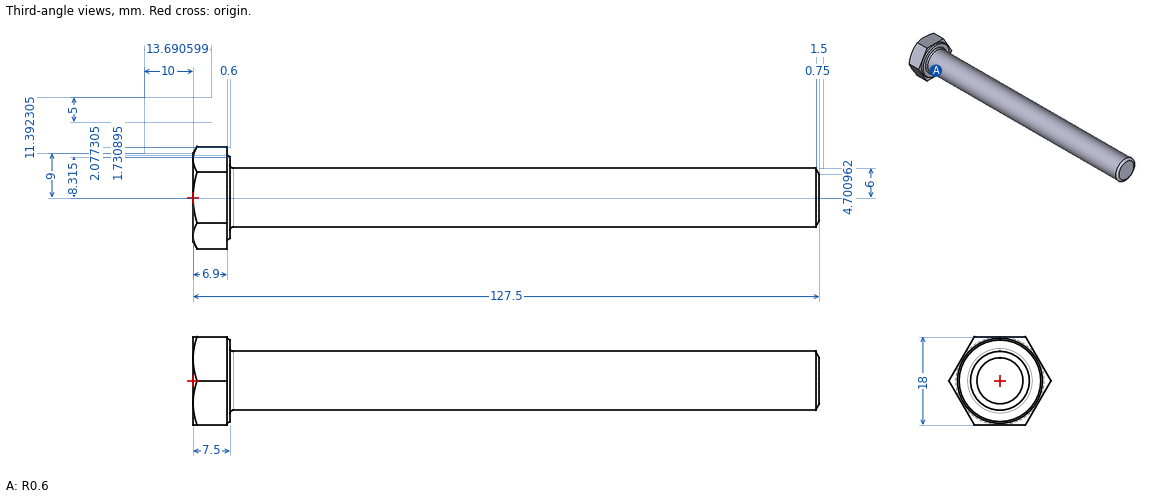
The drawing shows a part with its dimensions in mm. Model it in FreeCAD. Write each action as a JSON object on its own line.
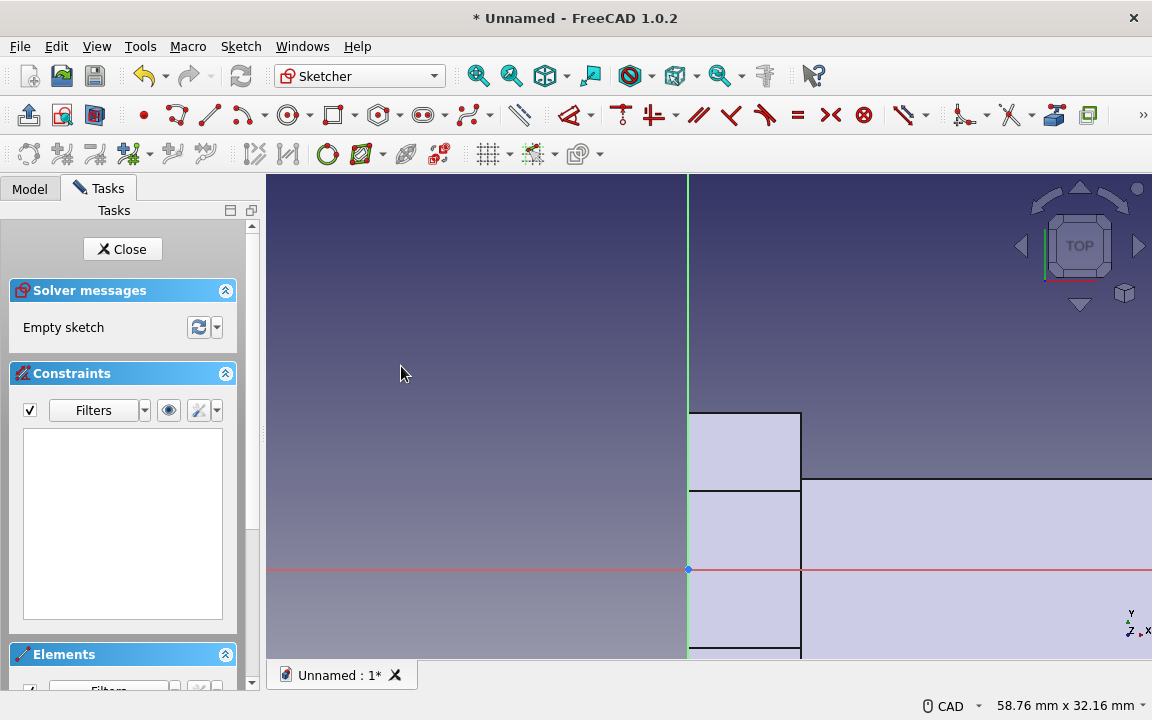
{"action": "left_click", "coordinate": [177, 116]}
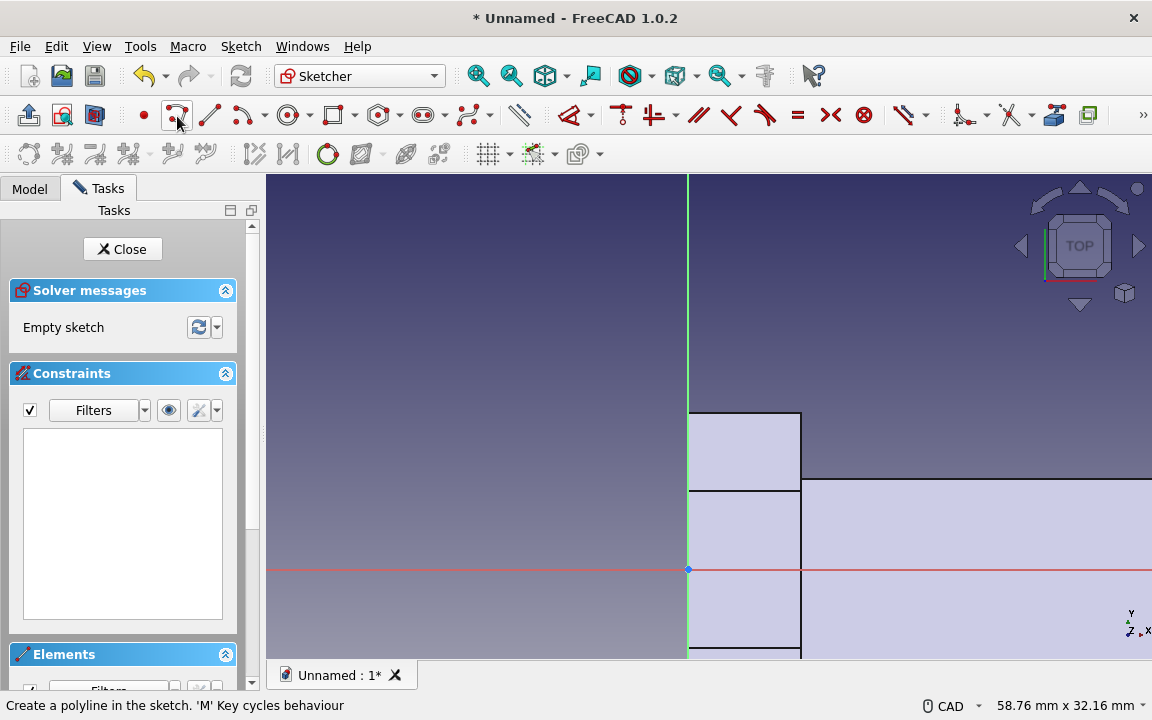
{"action": "left_click", "coordinate": [688, 434]}
{"action": "left_click", "coordinate": [744, 337]}
{"action": "left_click", "coordinate": [744, 262]}
{"action": "left_click", "coordinate": [537, 262]}
{"action": "left_click", "coordinate": [537, 434]}
{"action": "left_click", "coordinate": [688, 435]}
{"action": "key", "text": "Escape"}
{"action": "key", "text": "Escape"}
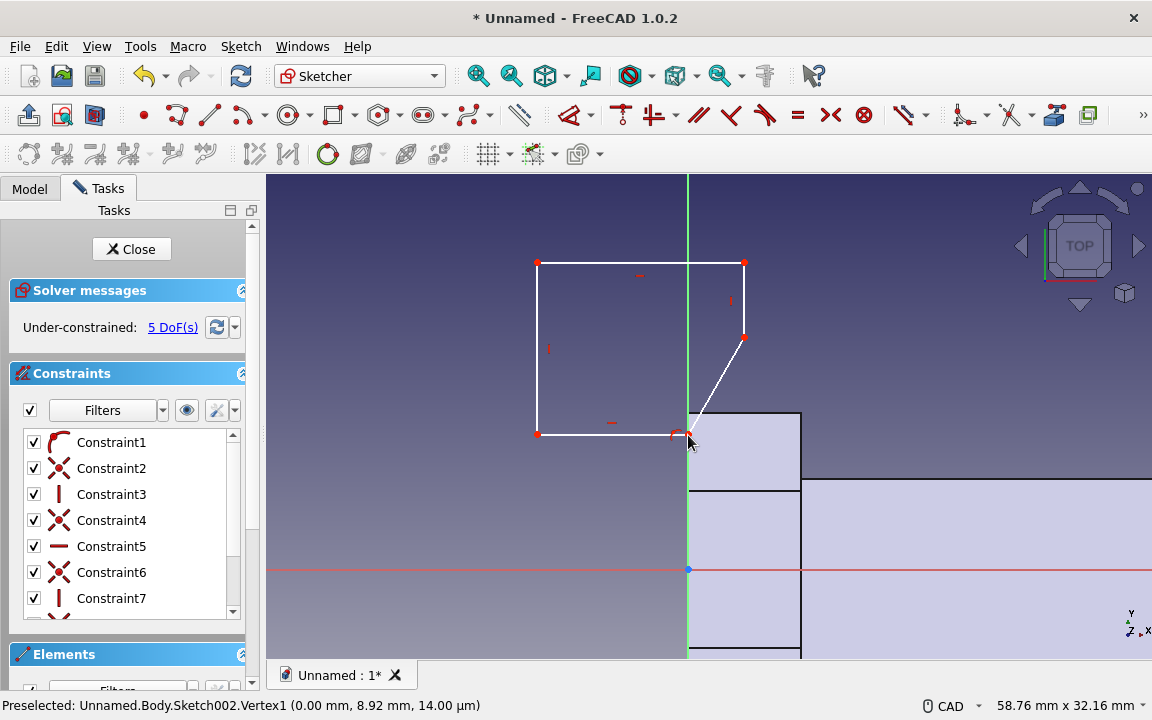
{"action": "left_click", "coordinate": [568, 116]}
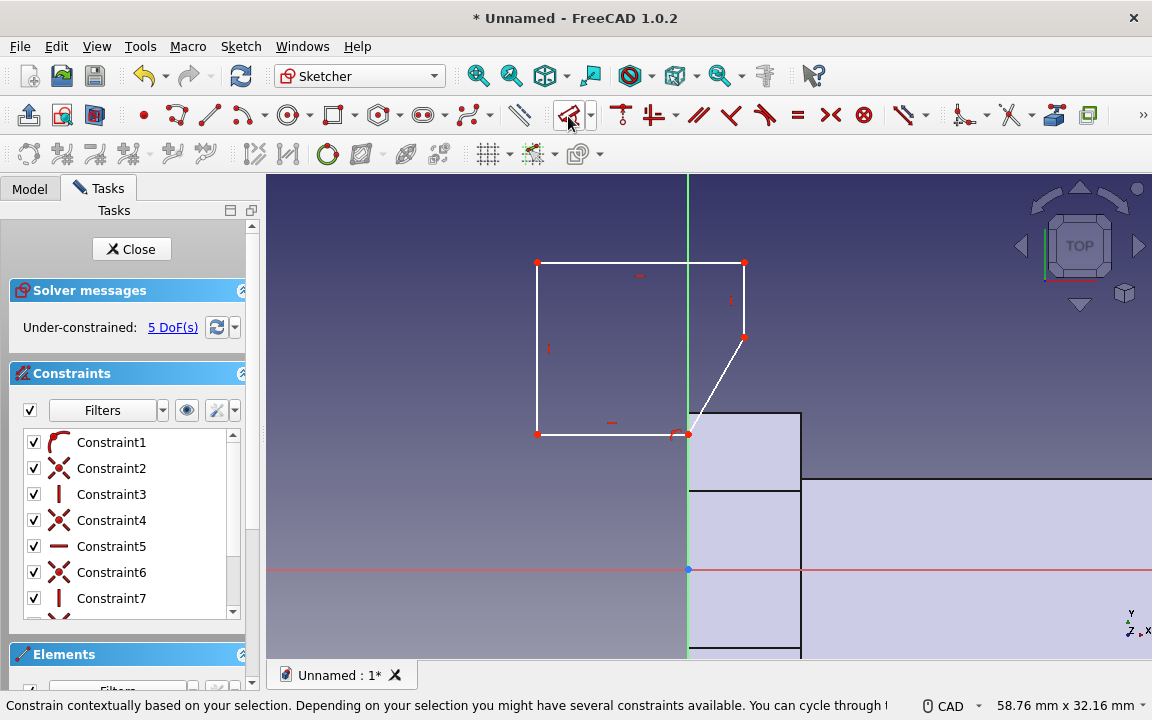
{"action": "left_click", "coordinate": [744, 315]}
{"action": "left_click", "coordinate": [778, 301]}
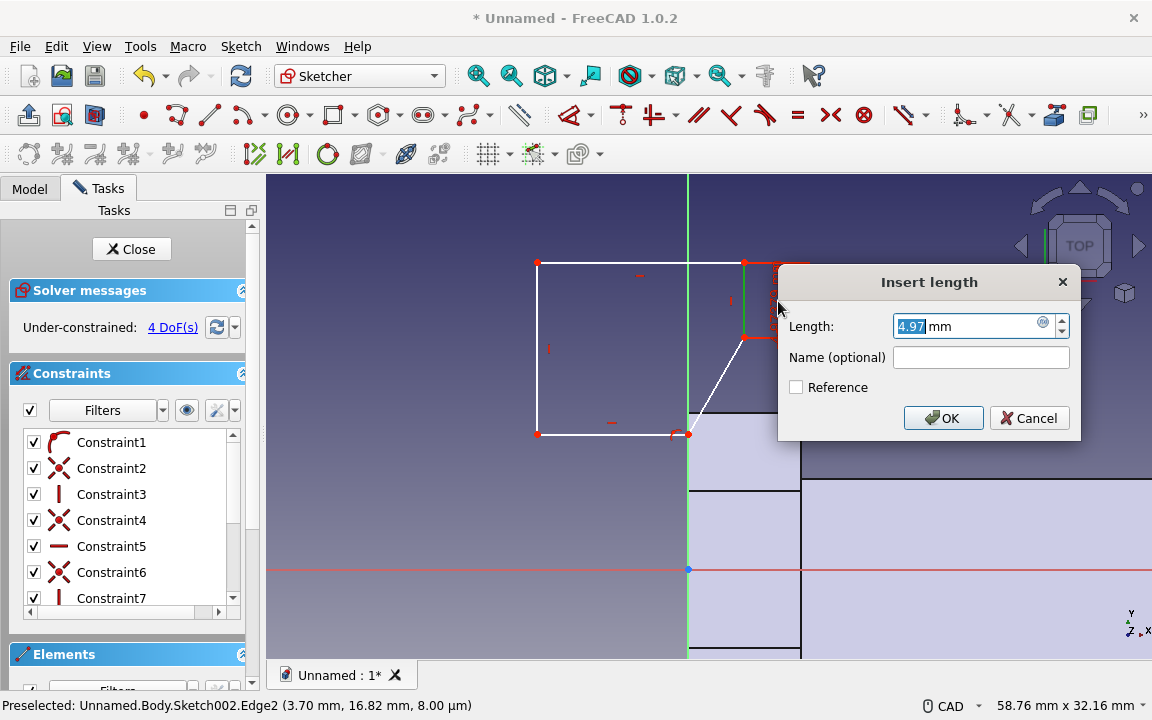
{"action": "type", "text": "5"}
{"action": "key", "text": "Return"}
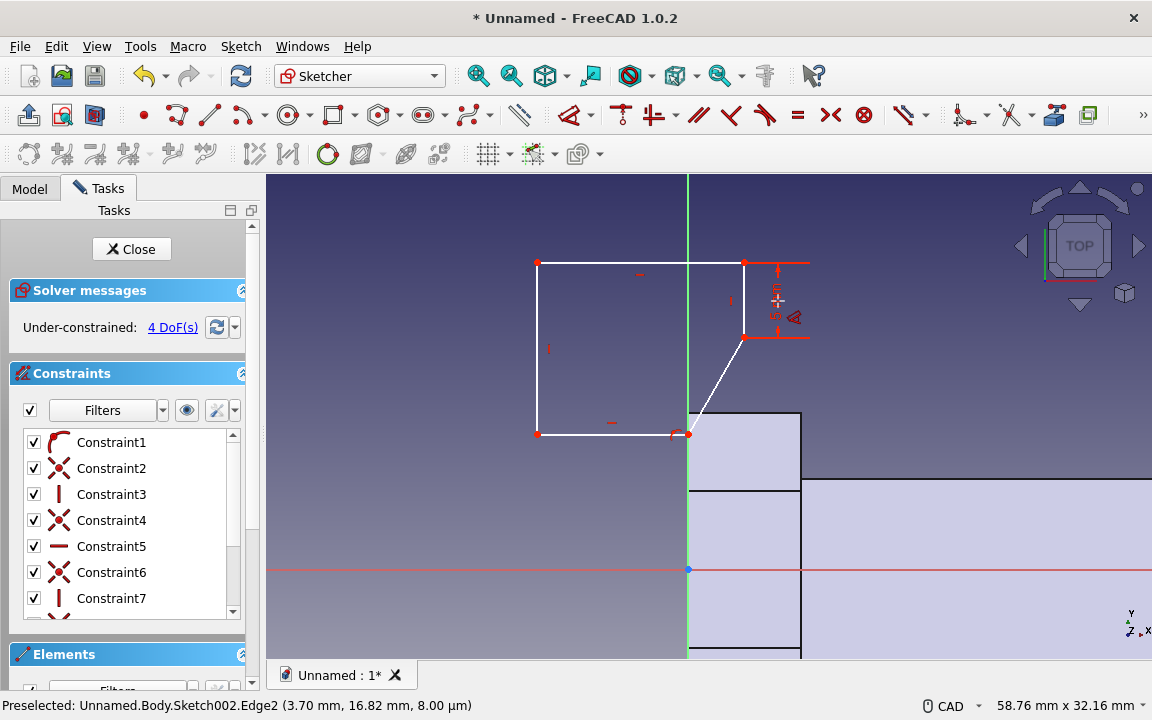
{"action": "left_click", "coordinate": [582, 435]}
{"action": "left_click", "coordinate": [613, 469]}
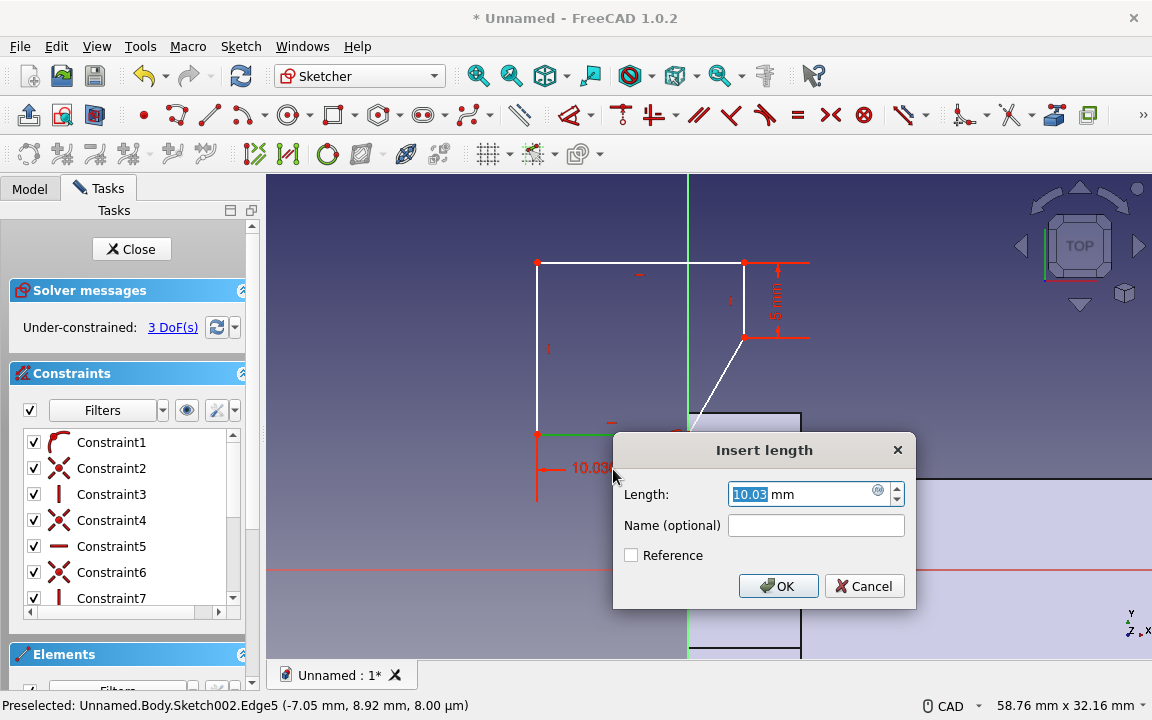
{"action": "type", "text": "10"}
{"action": "key", "text": "Return"}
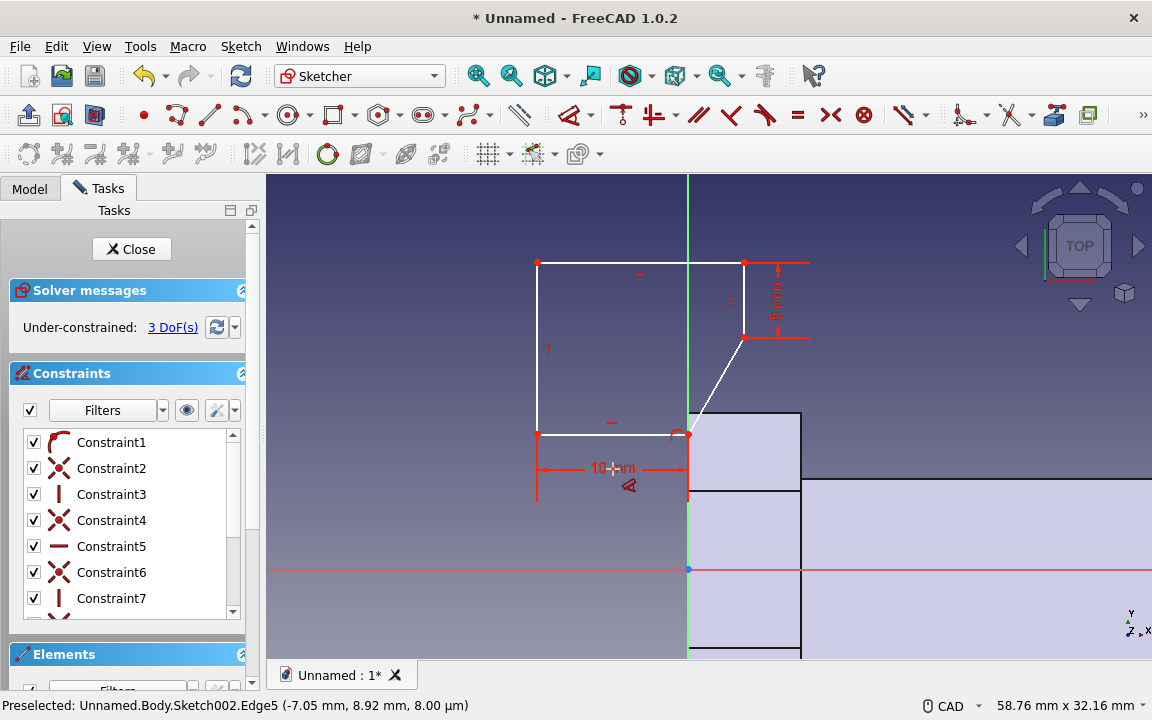
{"action": "left_click", "coordinate": [688, 435]}
{"action": "left_click", "coordinate": [722, 502]}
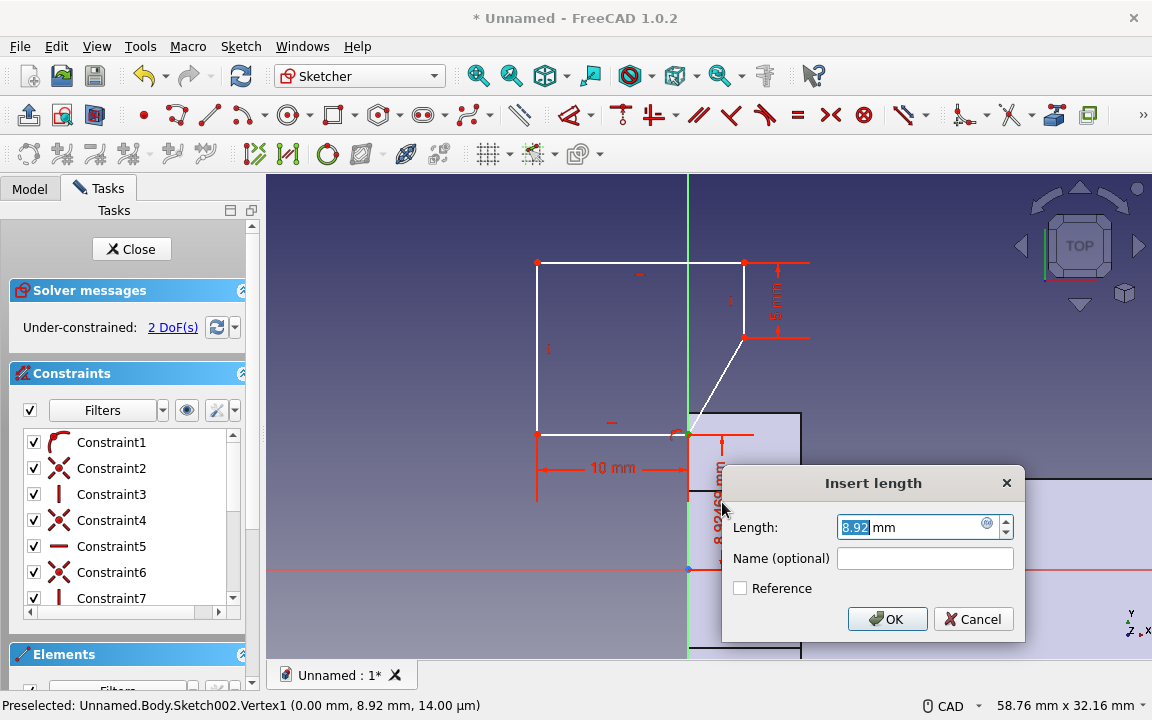
{"action": "type", "text": "9"}
{"action": "key", "text": "Return"}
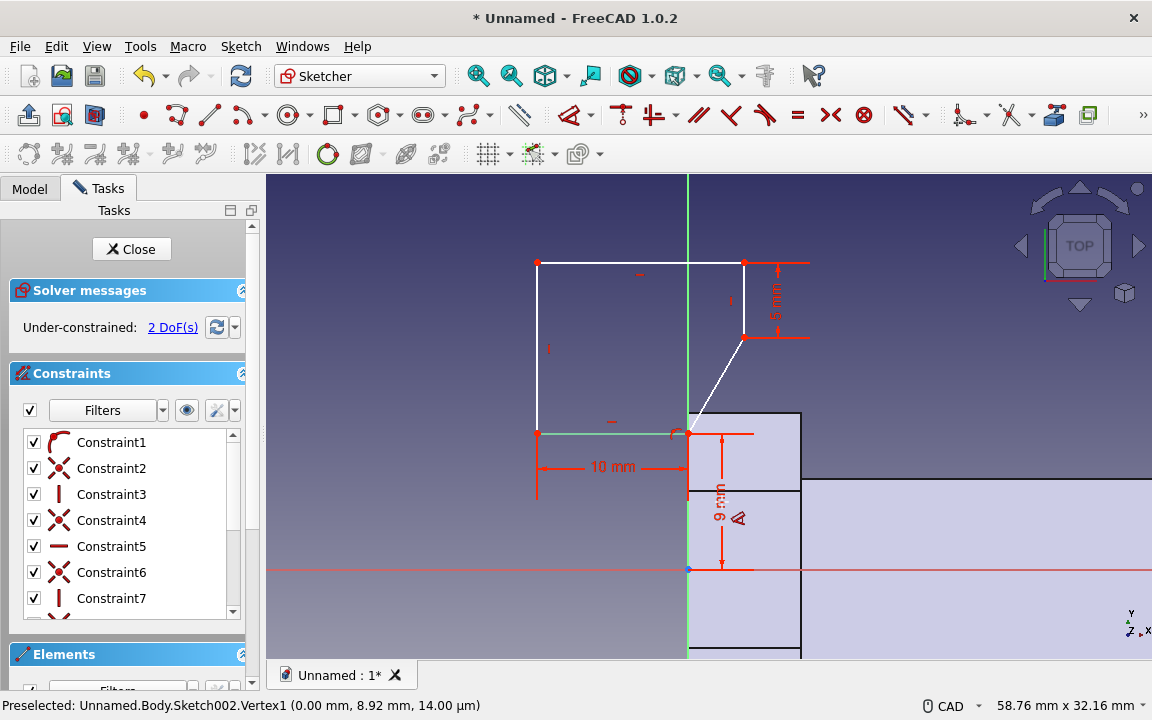
{"action": "left_click", "coordinate": [599, 263]}
{"action": "left_click", "coordinate": [641, 229]}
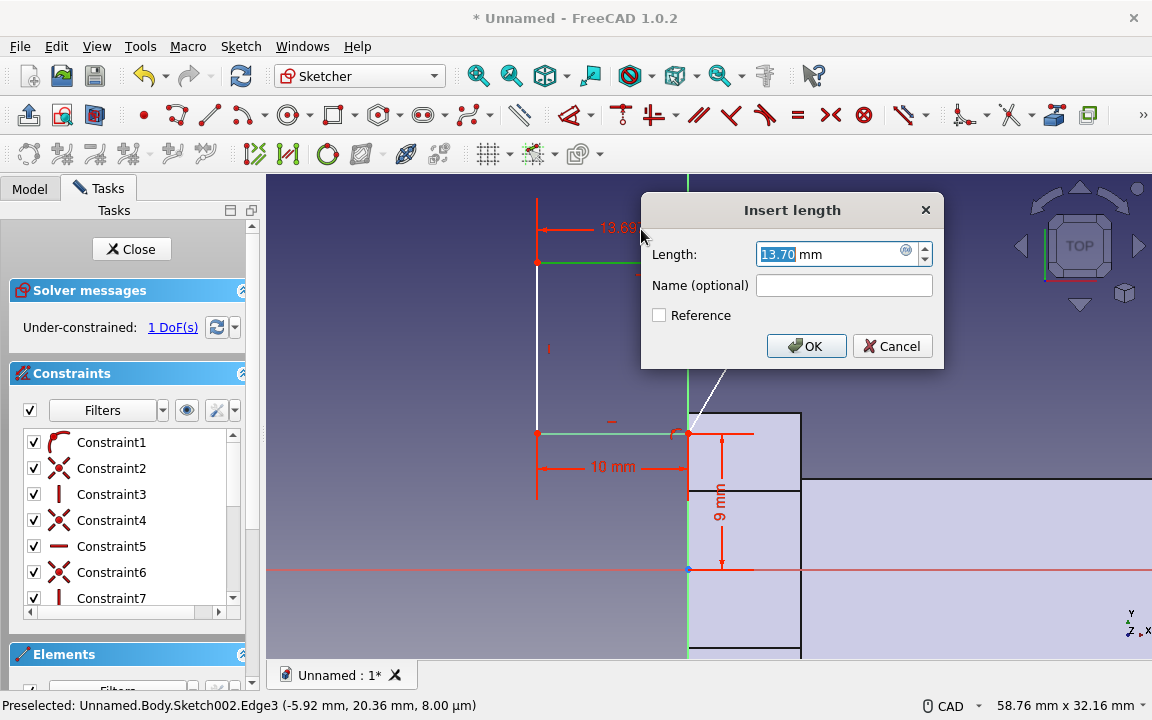
{"action": "type", "text": "13.690599"}
{"action": "key", "text": "Return"}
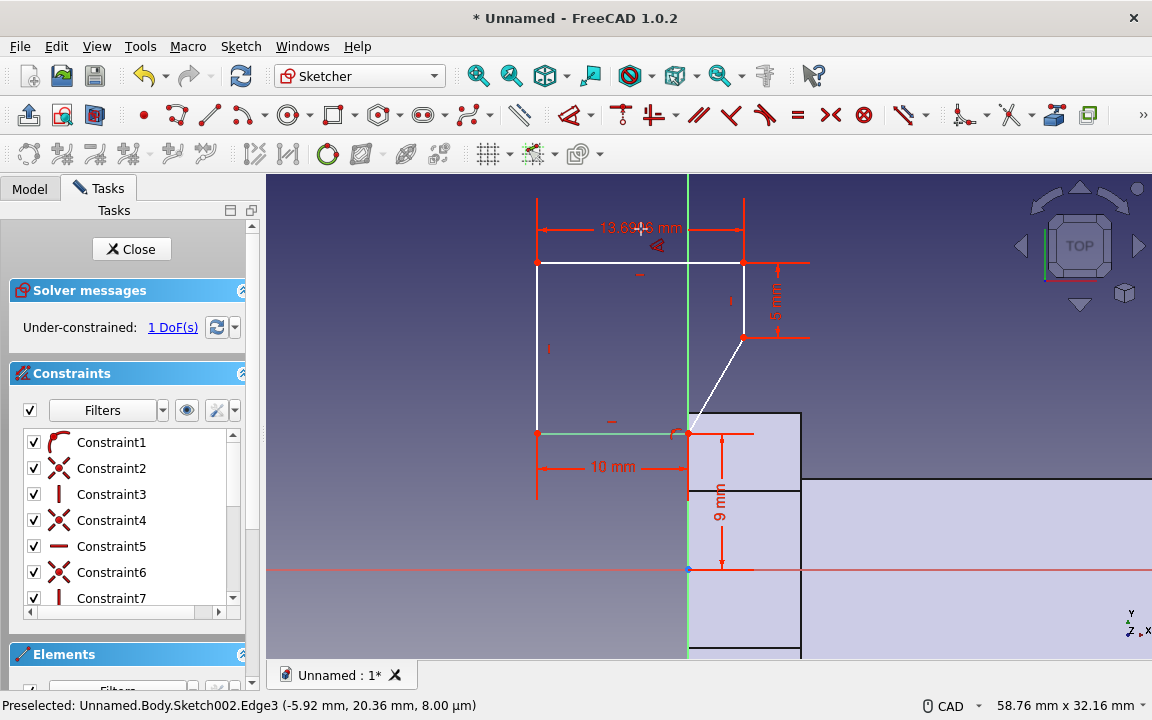
{"action": "left_click", "coordinate": [537, 314]}
{"action": "left_click", "coordinate": [503, 348]}